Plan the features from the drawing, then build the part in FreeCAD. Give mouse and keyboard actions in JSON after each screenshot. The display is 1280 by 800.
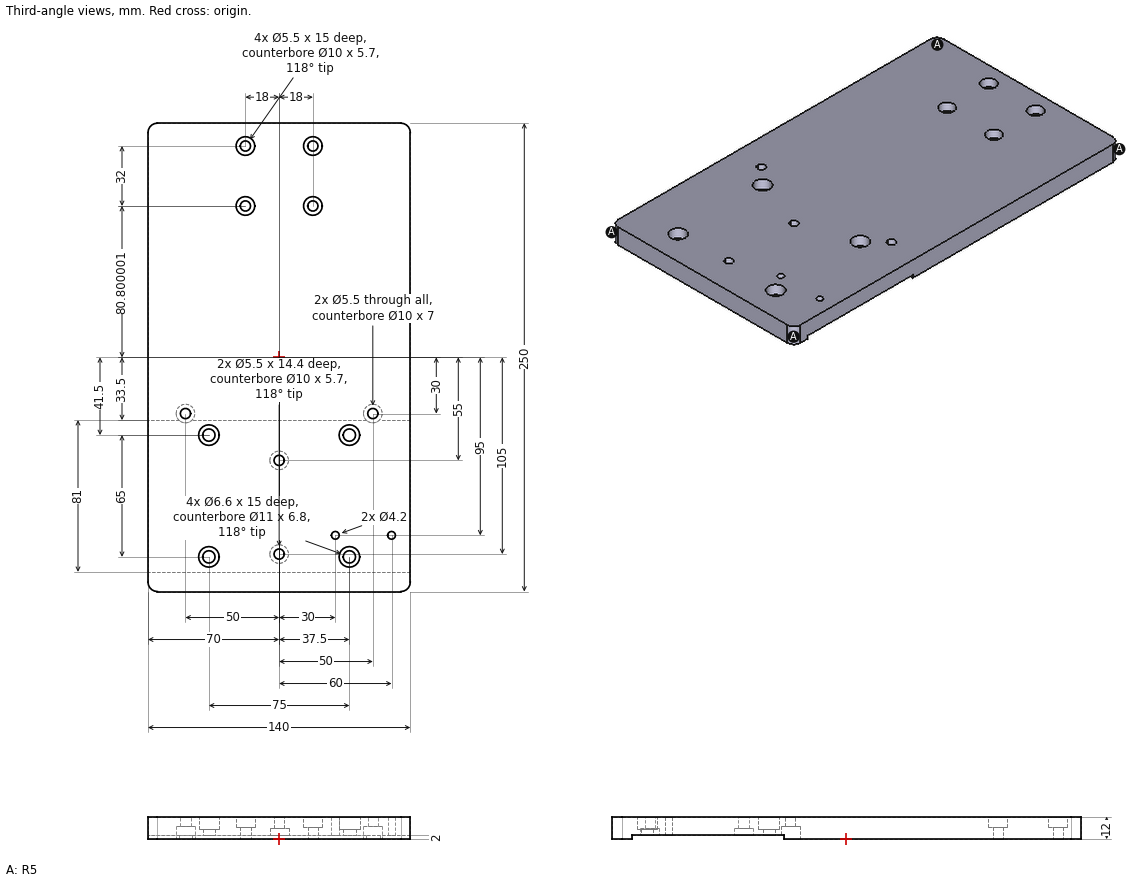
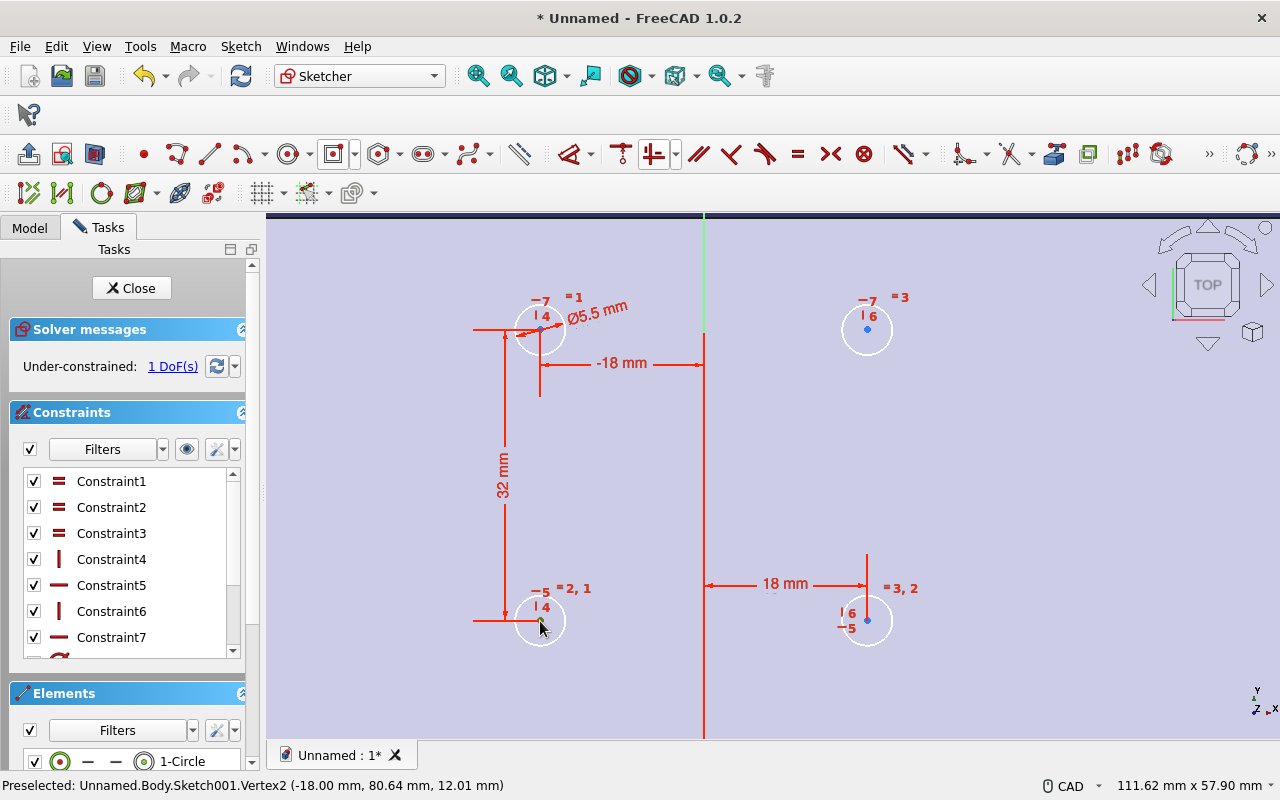
{"action": "key", "text": "i"}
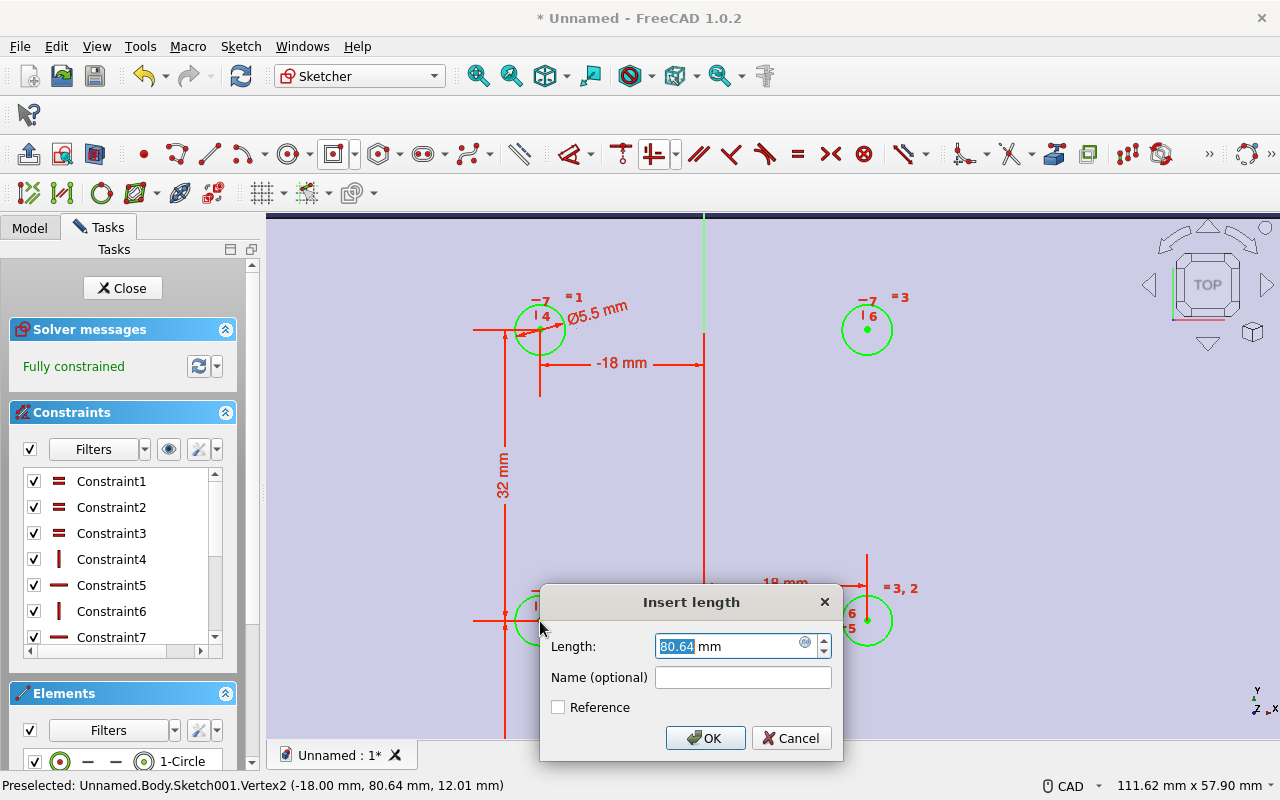
{"action": "type", "text": "80.800001"}
{"action": "key", "text": "Return"}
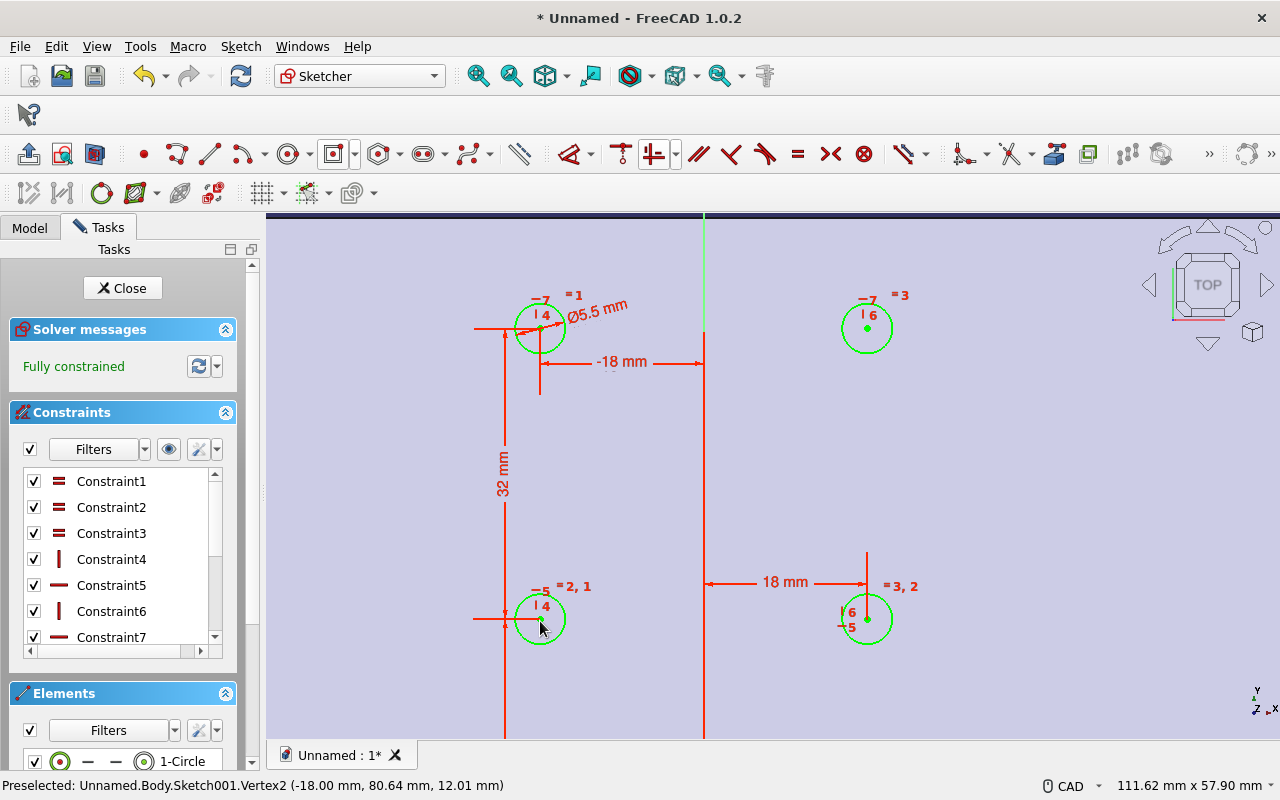
{"action": "left_click", "coordinate": [123, 288]}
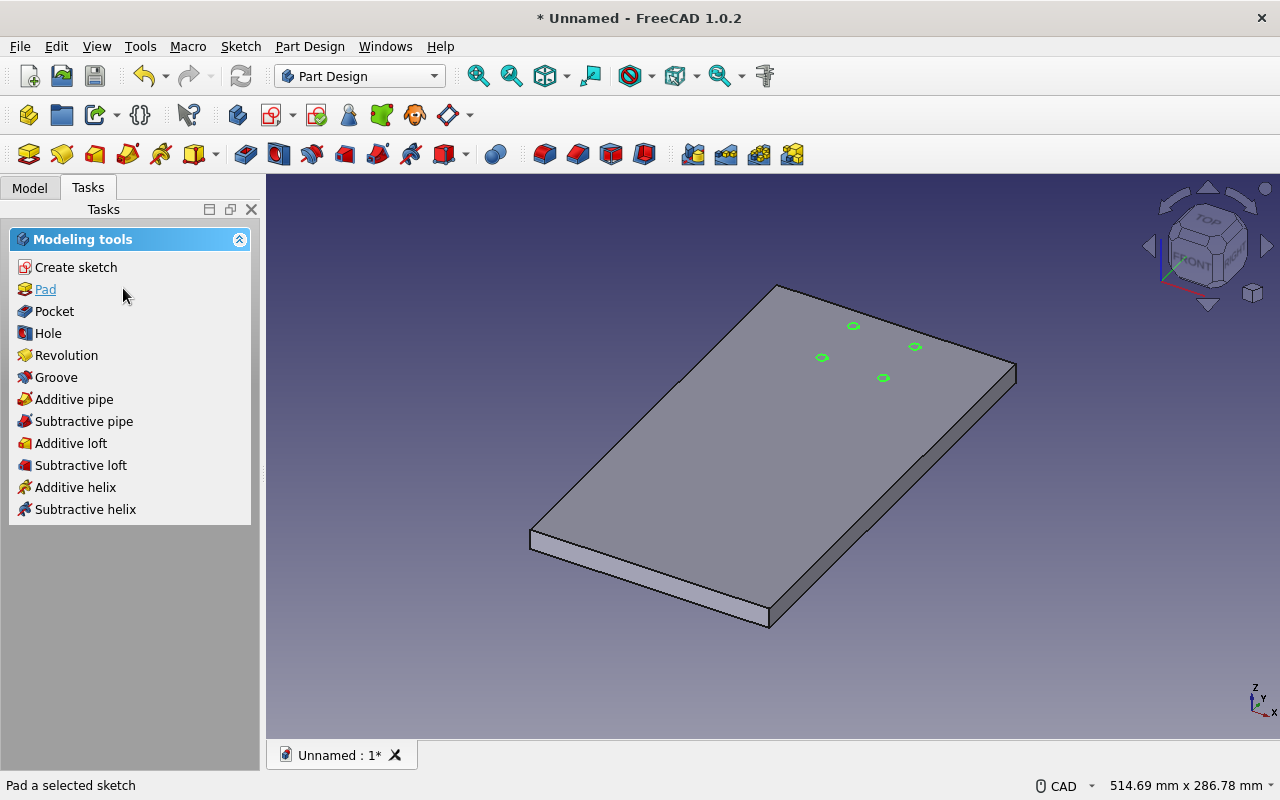
{"action": "left_click", "coordinate": [279, 154]}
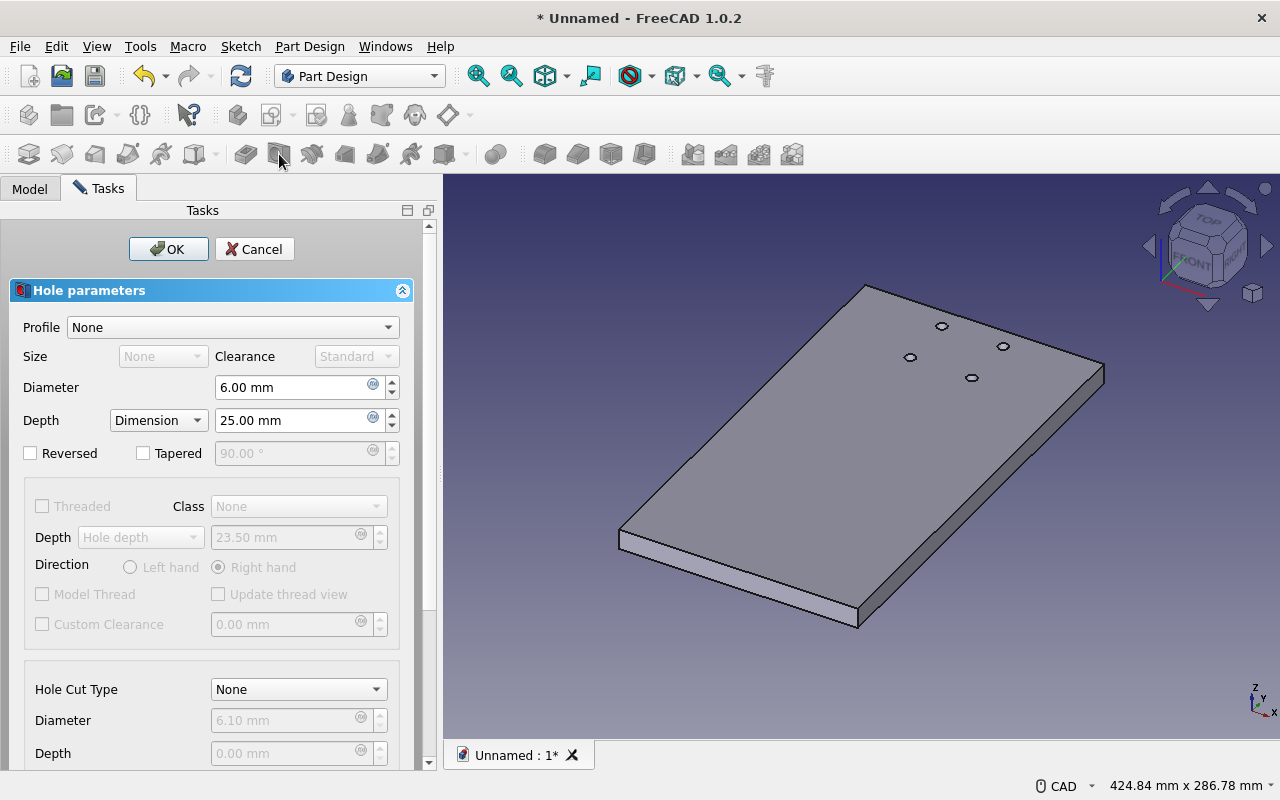
{"action": "triple_click", "coordinate": [300, 388]}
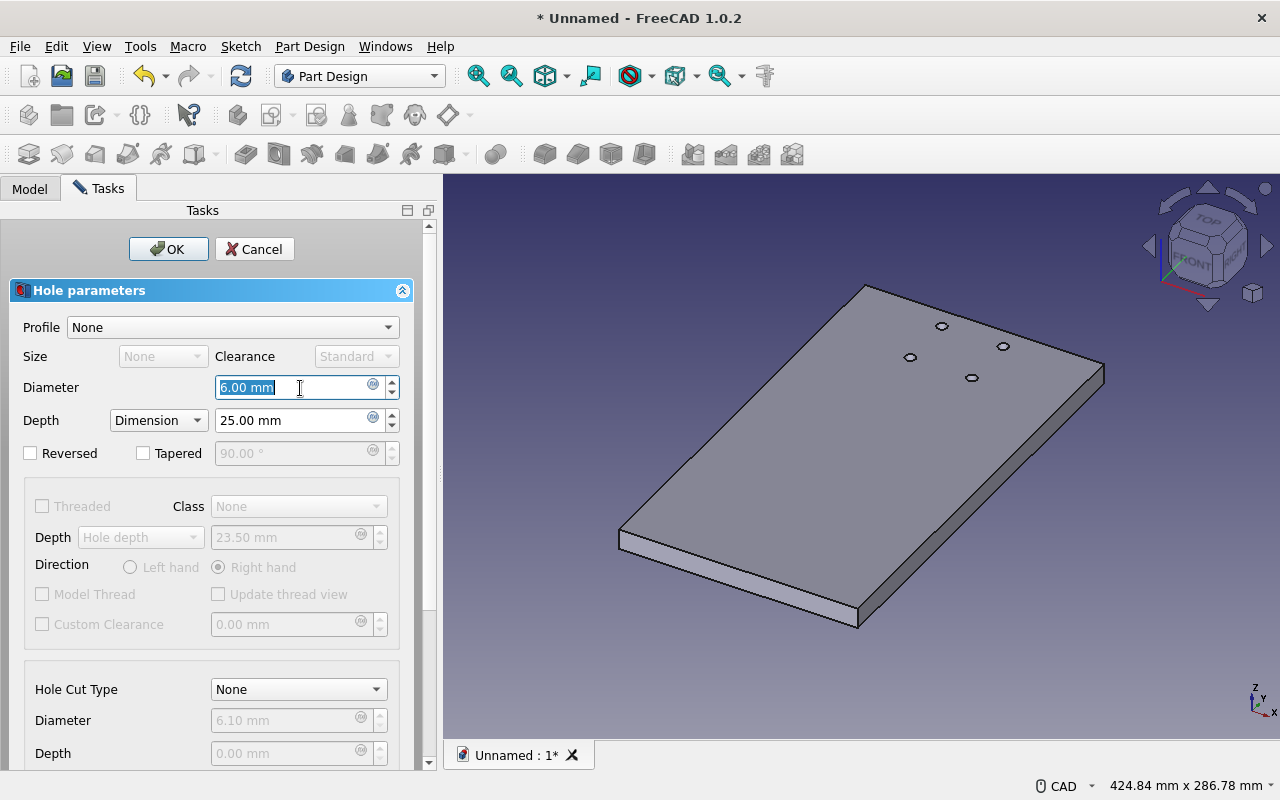
{"action": "type", "text": "5.5"}
{"action": "key", "text": "Tab"}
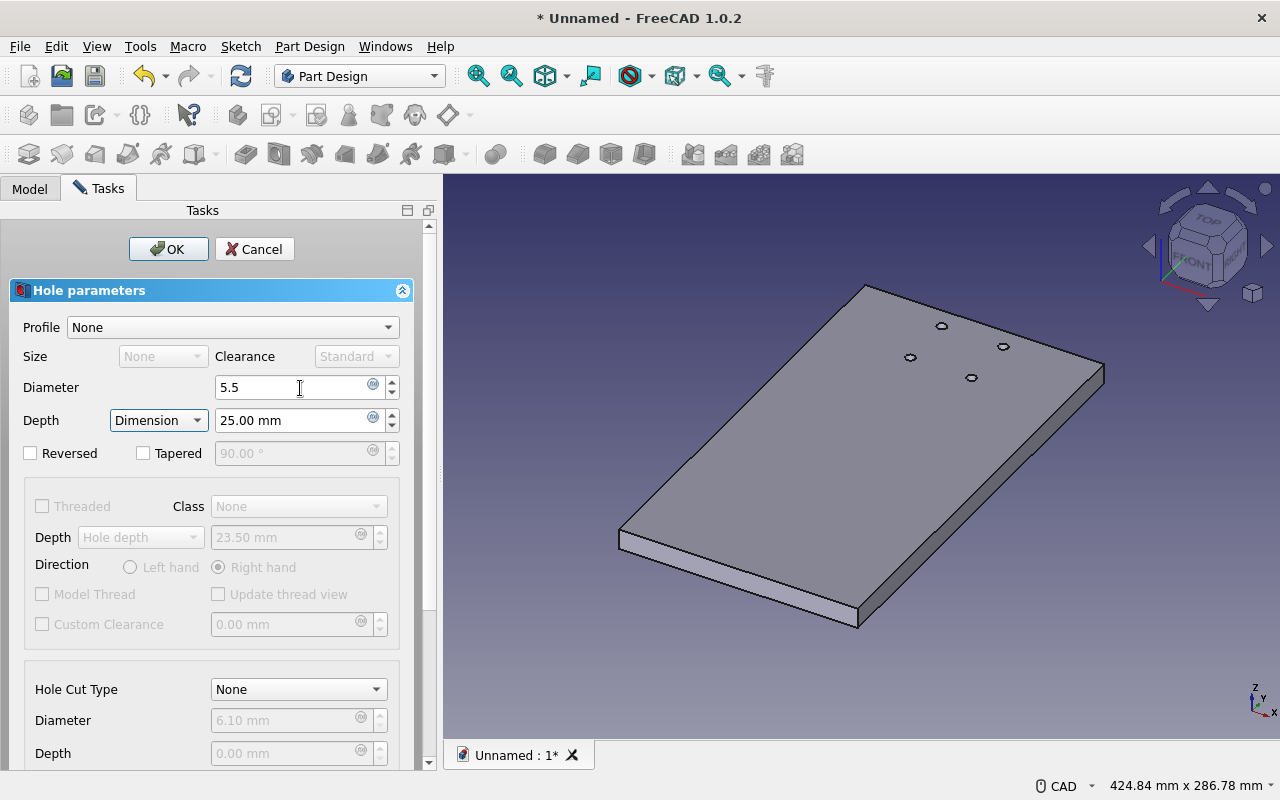
{"action": "triple_click", "coordinate": [300, 420]}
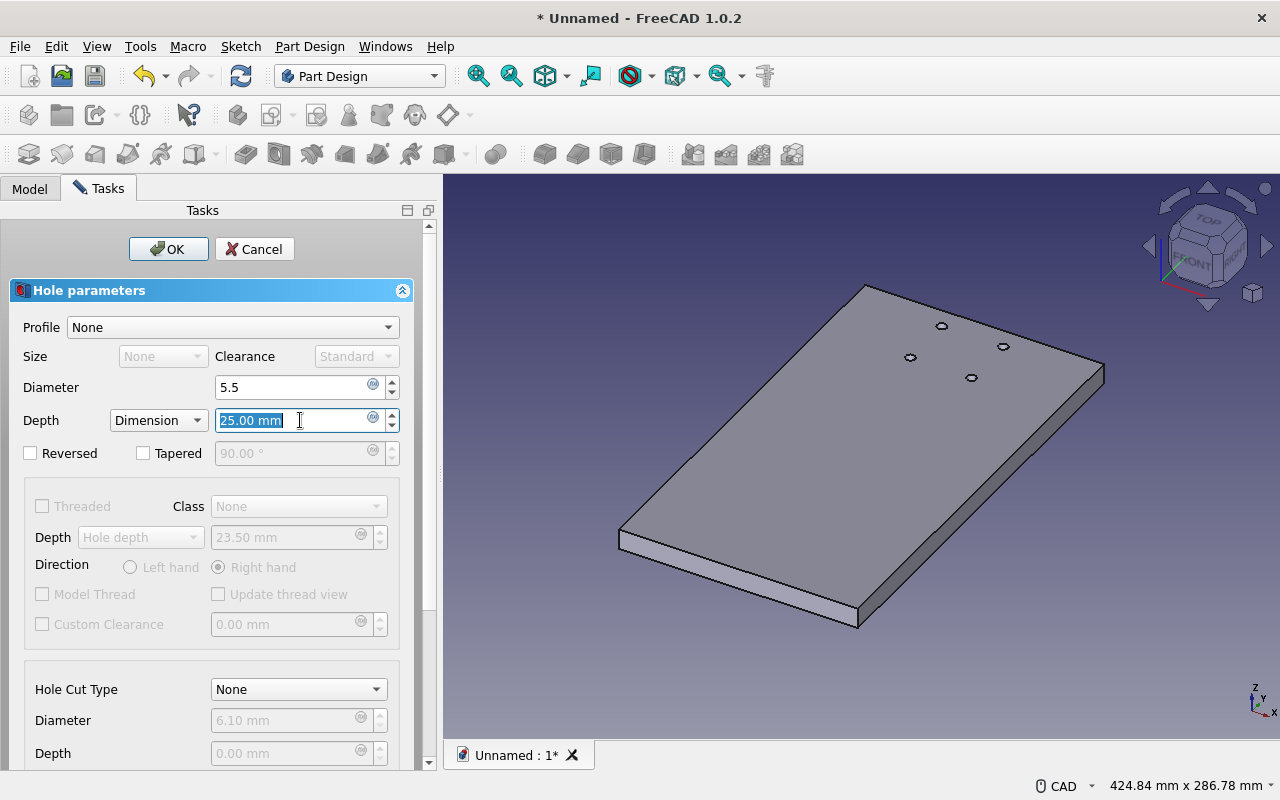
{"action": "type", "text": "15"}
{"action": "key", "text": "Tab"}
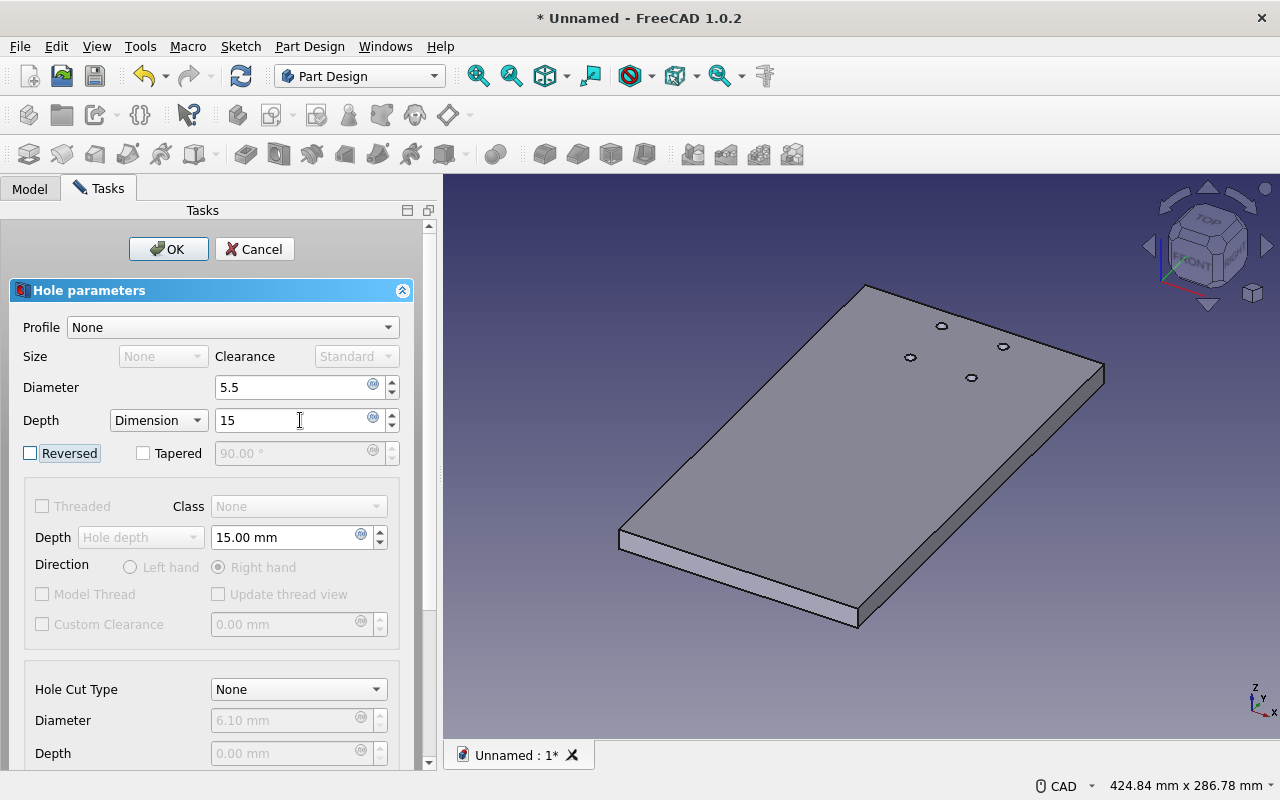
{"action": "left_click", "coordinate": [300, 690]}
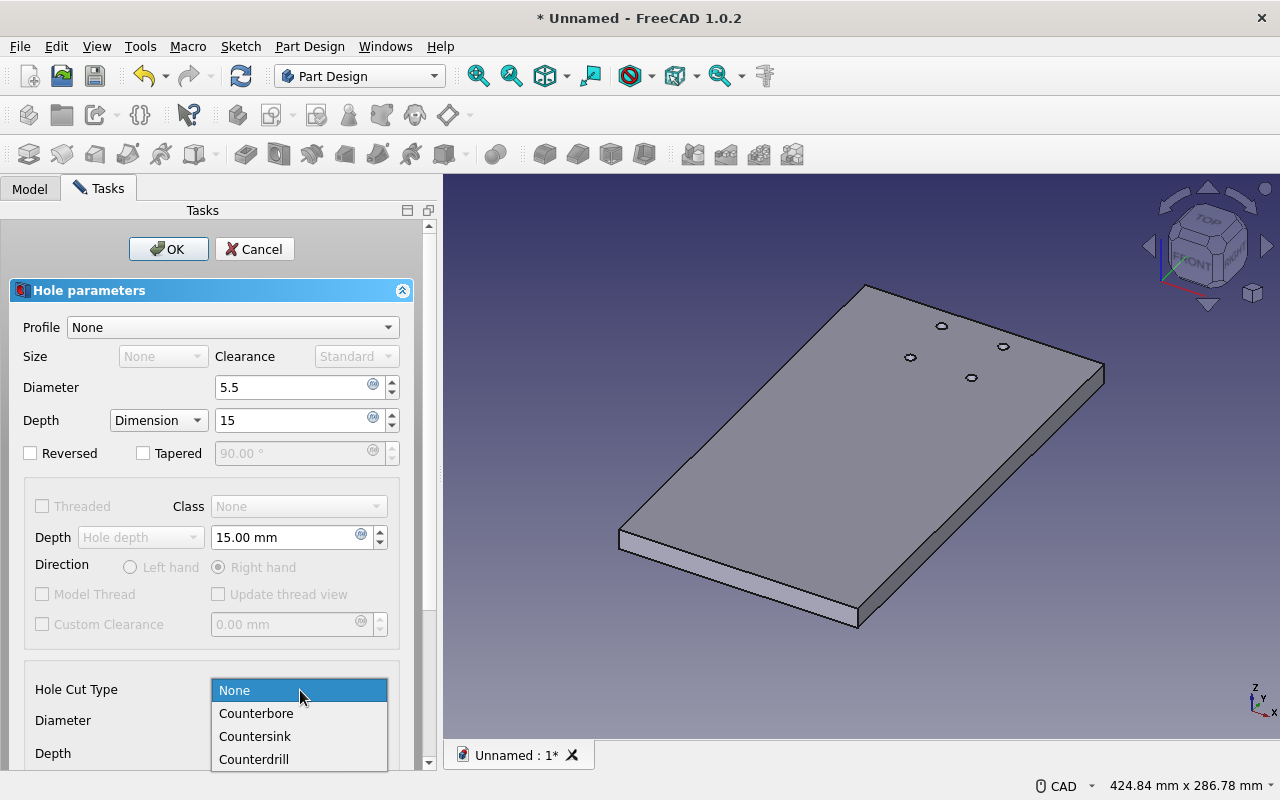
{"action": "left_click", "coordinate": [298, 714]}